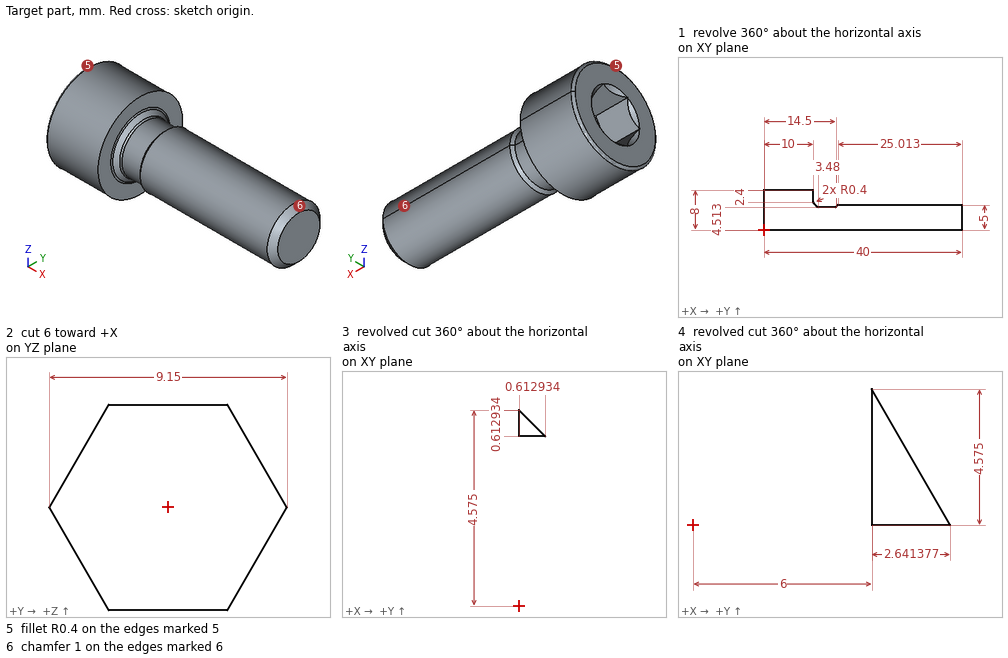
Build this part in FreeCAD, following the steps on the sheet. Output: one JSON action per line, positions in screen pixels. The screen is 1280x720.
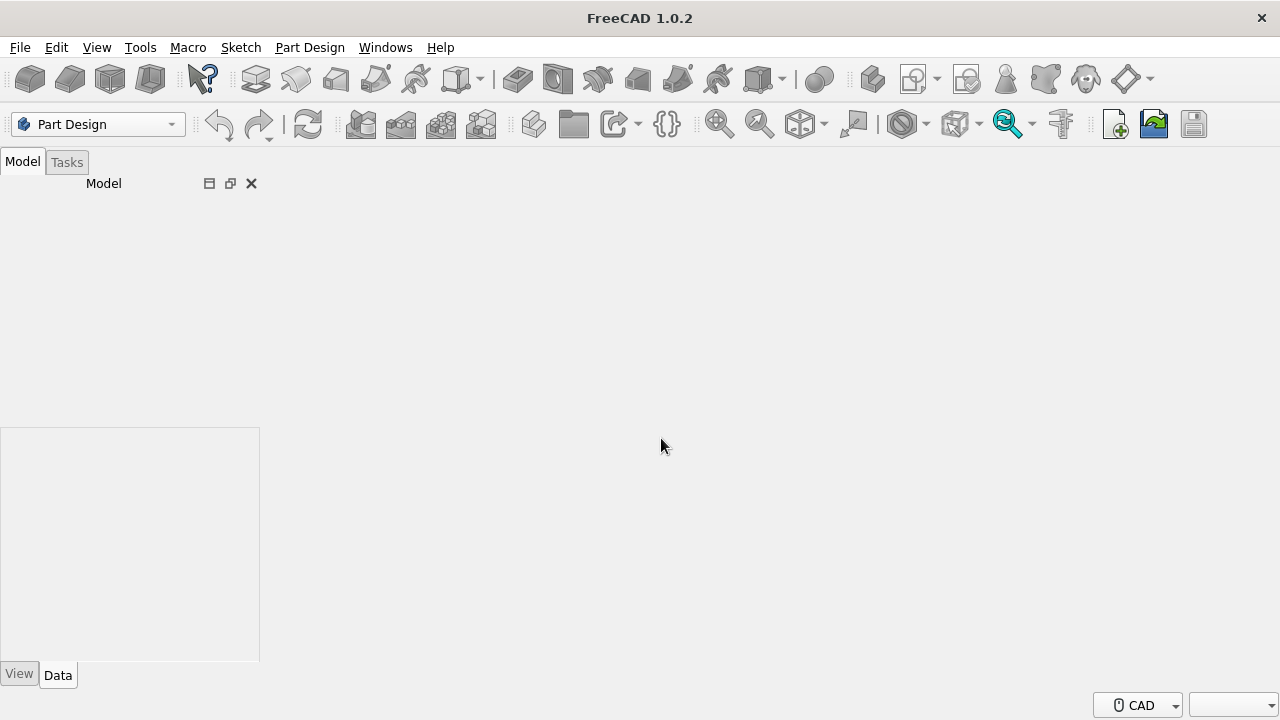
{"action": "left_click", "coordinate": [1114, 124]}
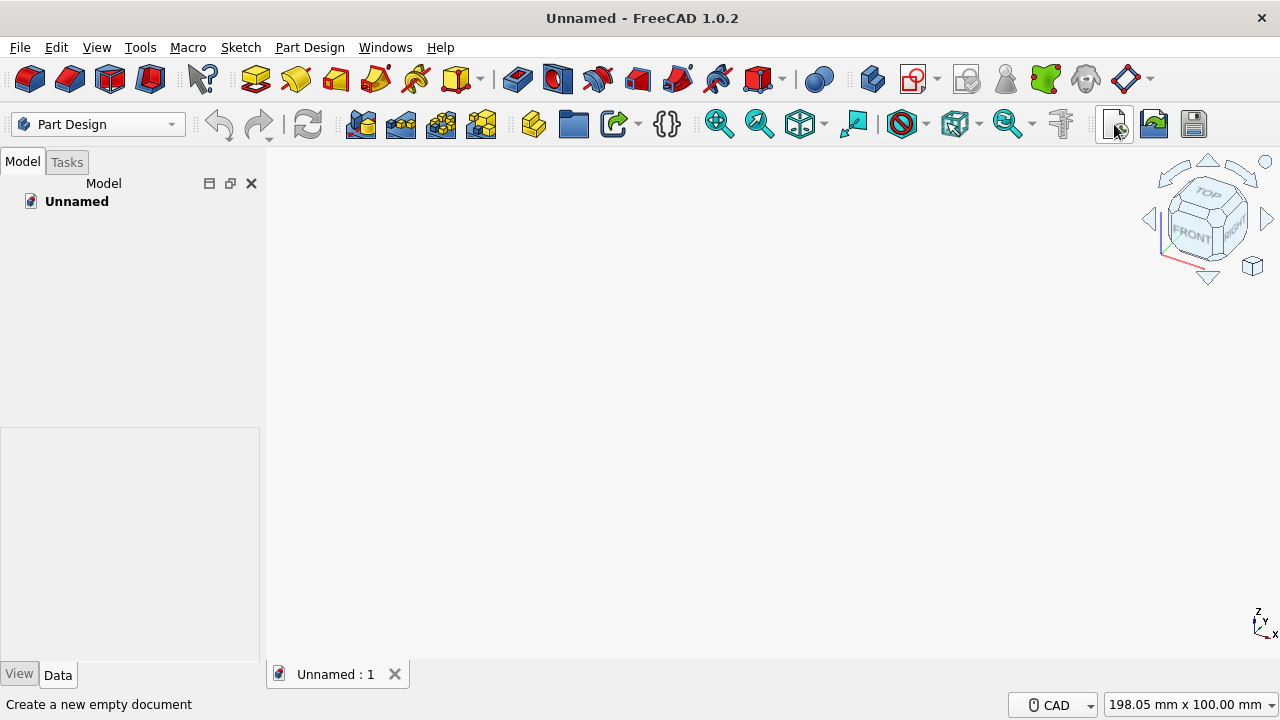
{"action": "left_click", "coordinate": [914, 80]}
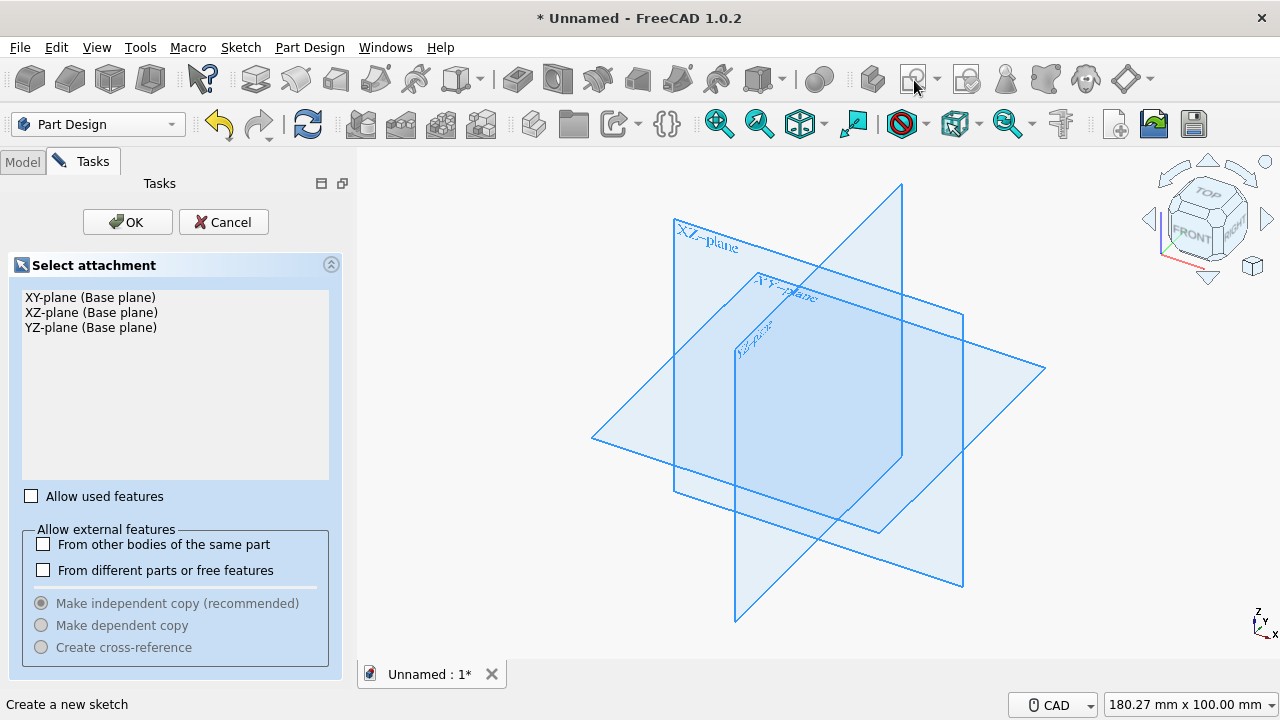
{"action": "left_click", "coordinate": [82, 298]}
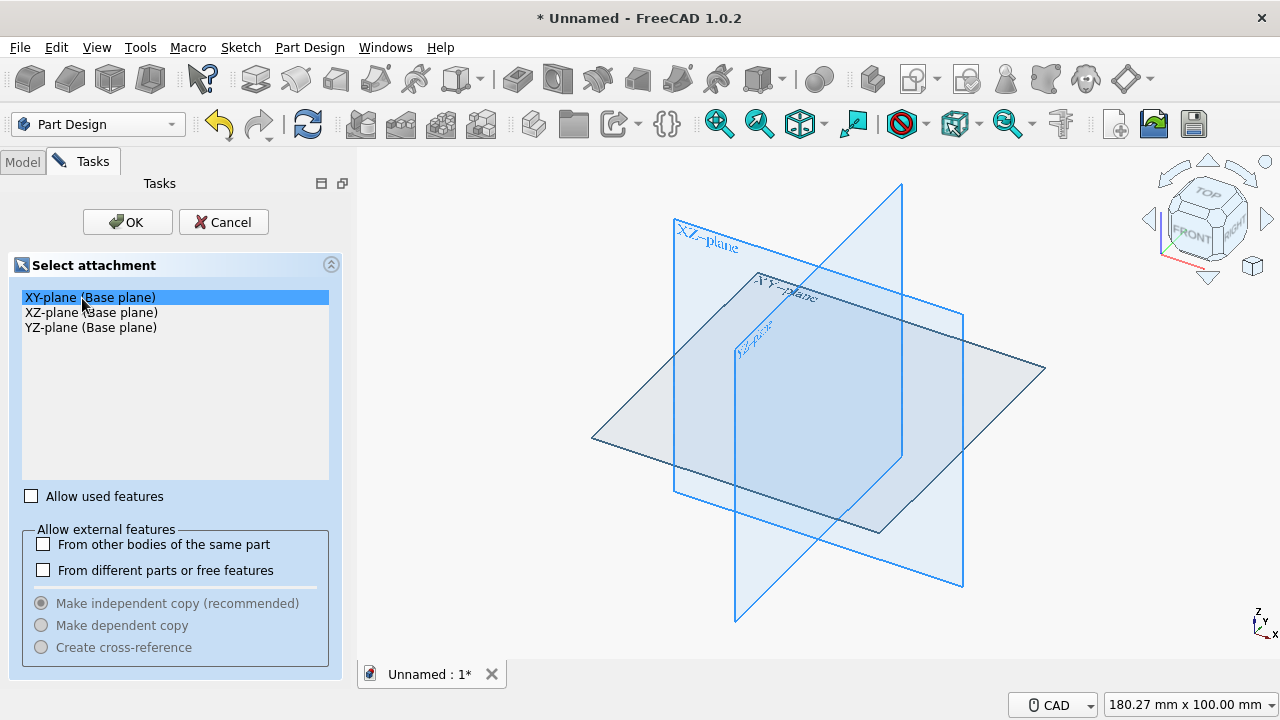
{"action": "left_click", "coordinate": [128, 222]}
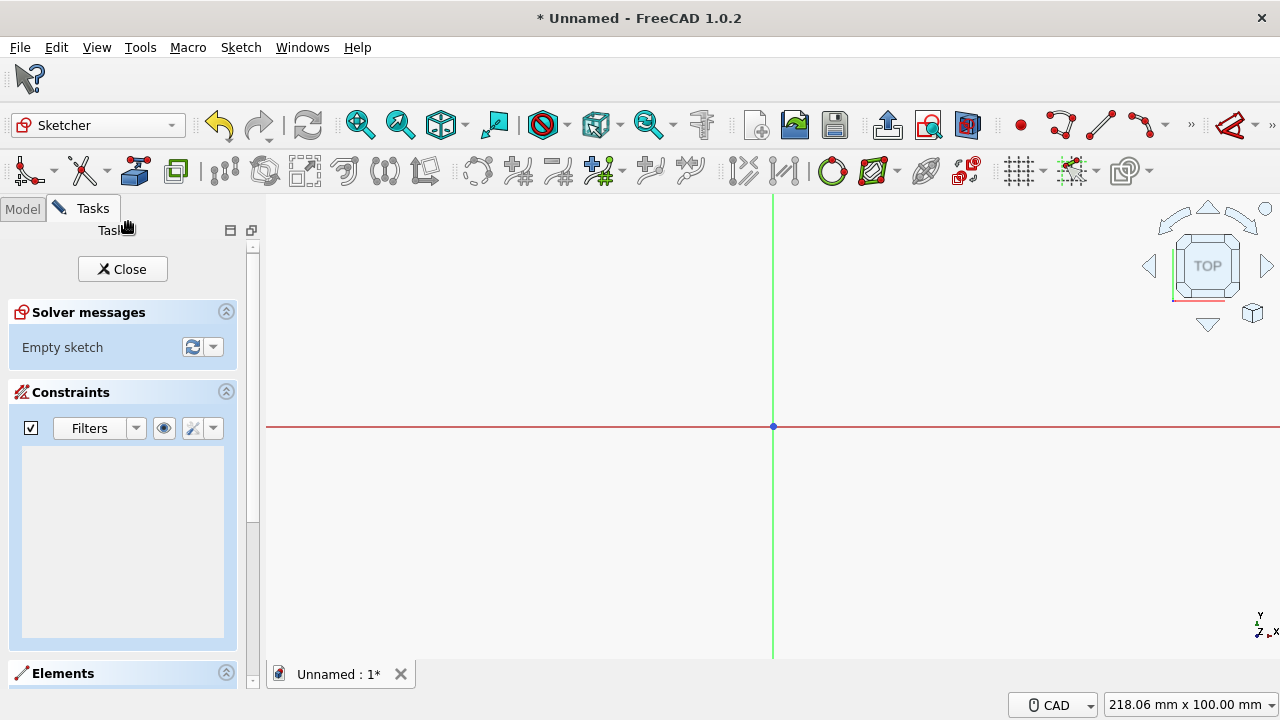
{"action": "scroll", "coordinate": [936, 400], "scroll_direction": "up", "scroll_amount": 6}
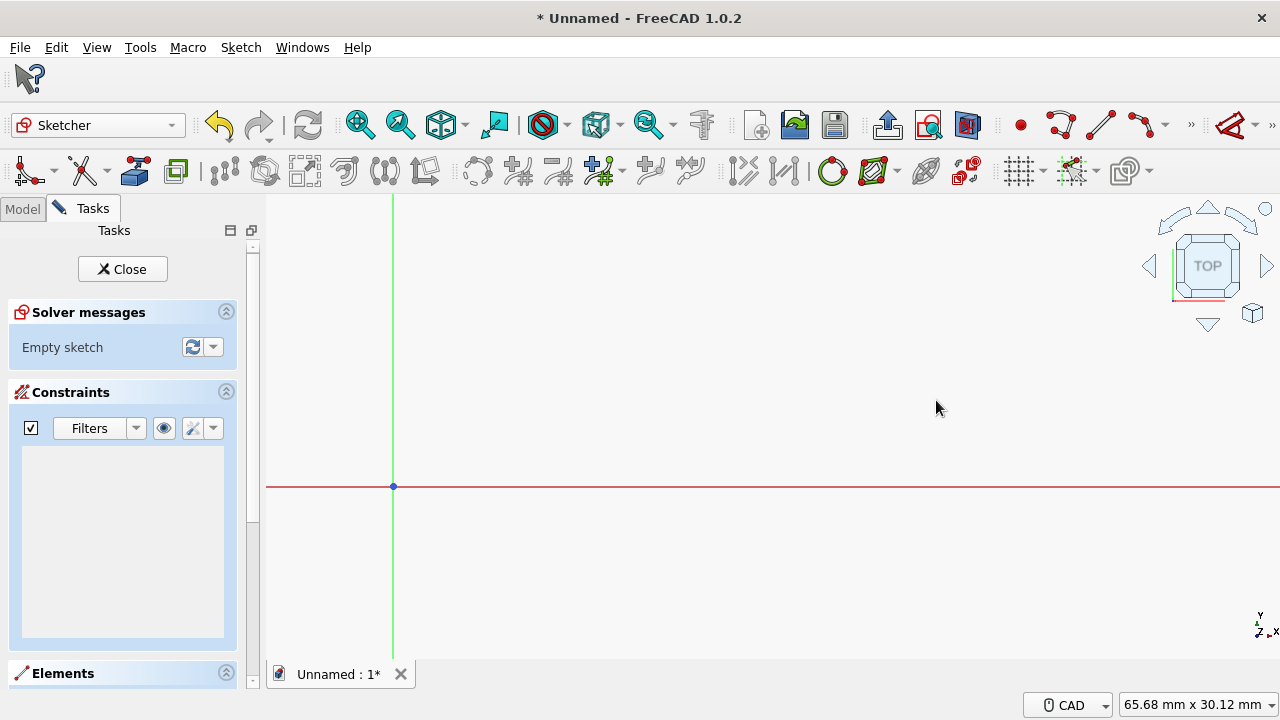
{"action": "left_click", "coordinate": [1102, 126]}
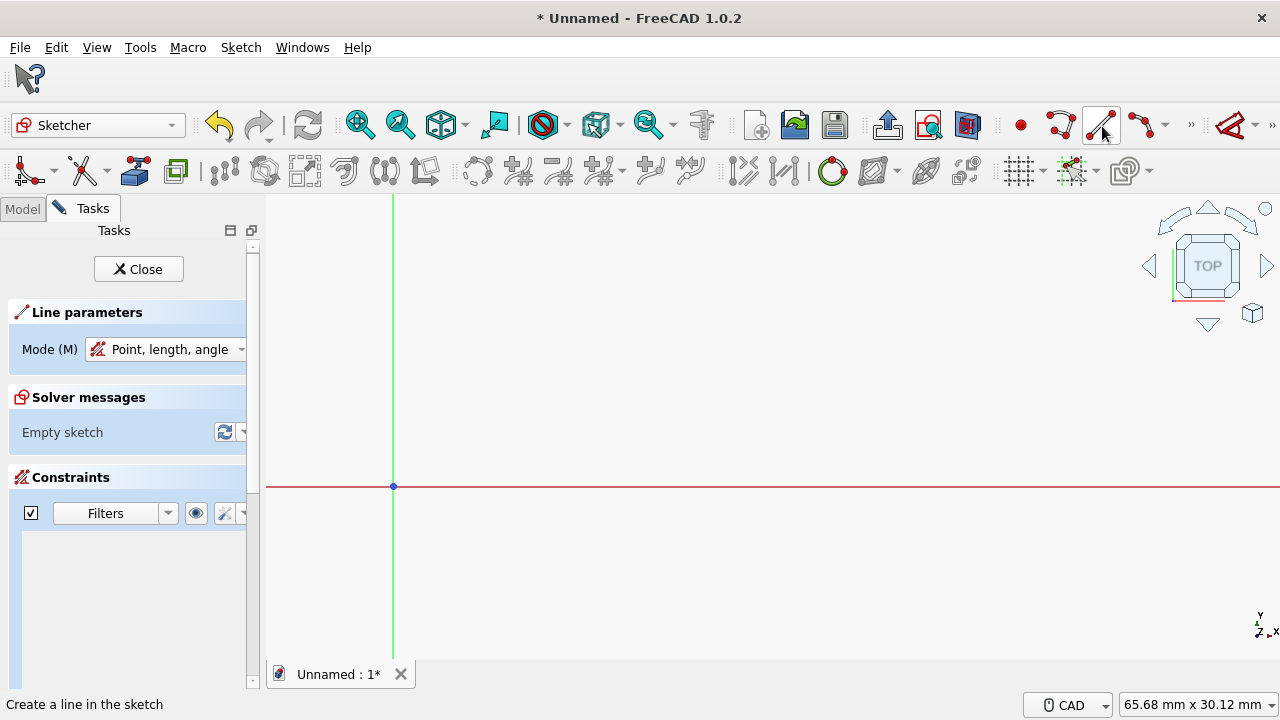
{"action": "left_click", "coordinate": [559, 415]}
{"action": "left_click", "coordinate": [549, 405]}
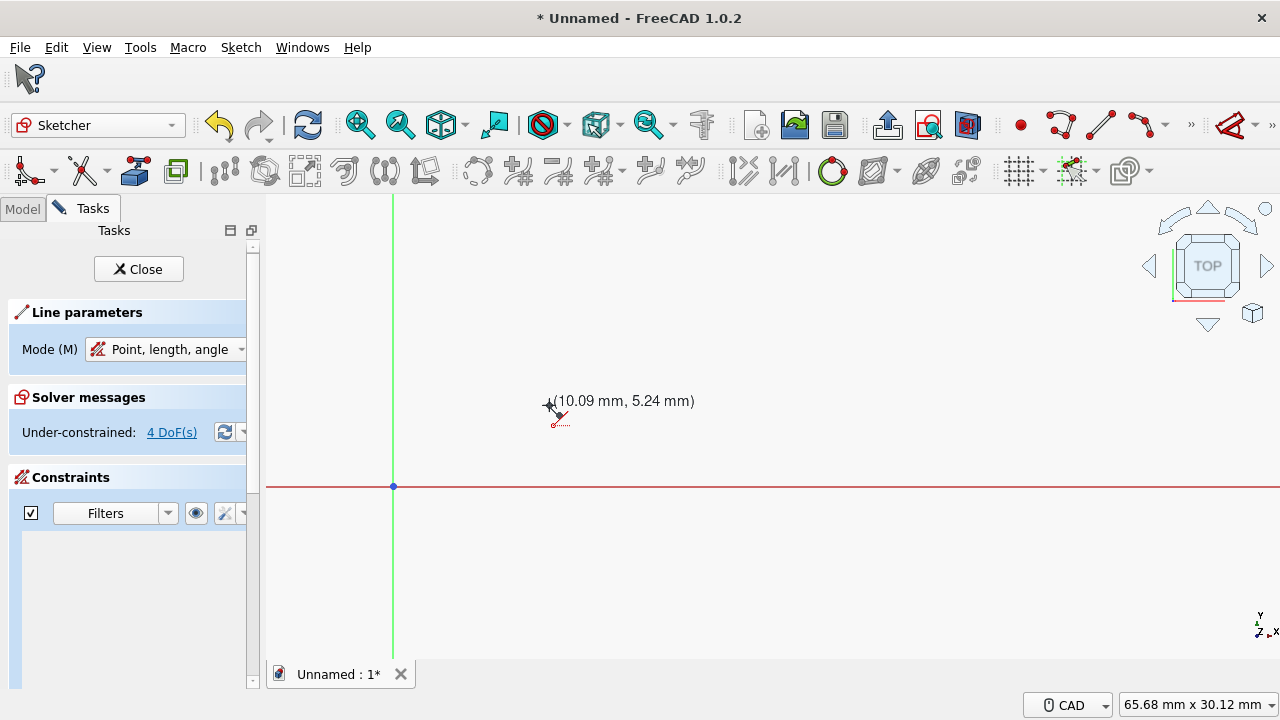
{"action": "left_click", "coordinate": [1062, 126]}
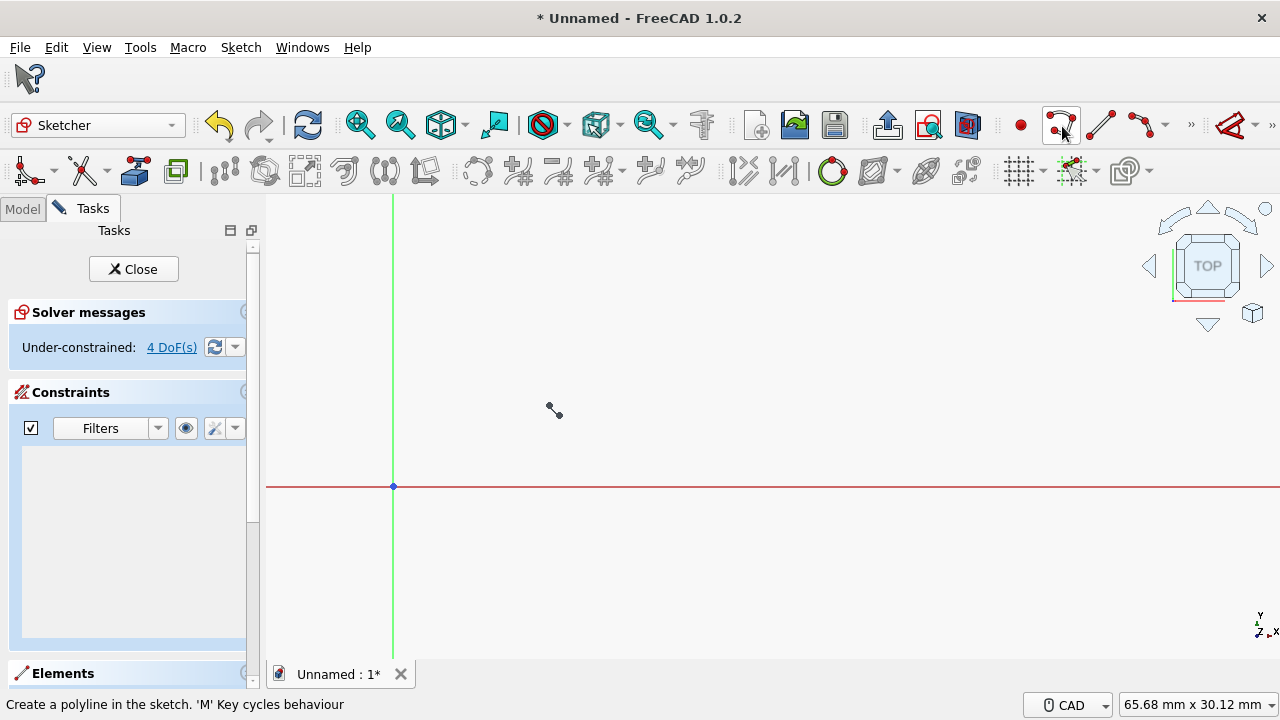
{"action": "scroll", "coordinate": [548, 400], "scroll_direction": "up", "scroll_amount": 7}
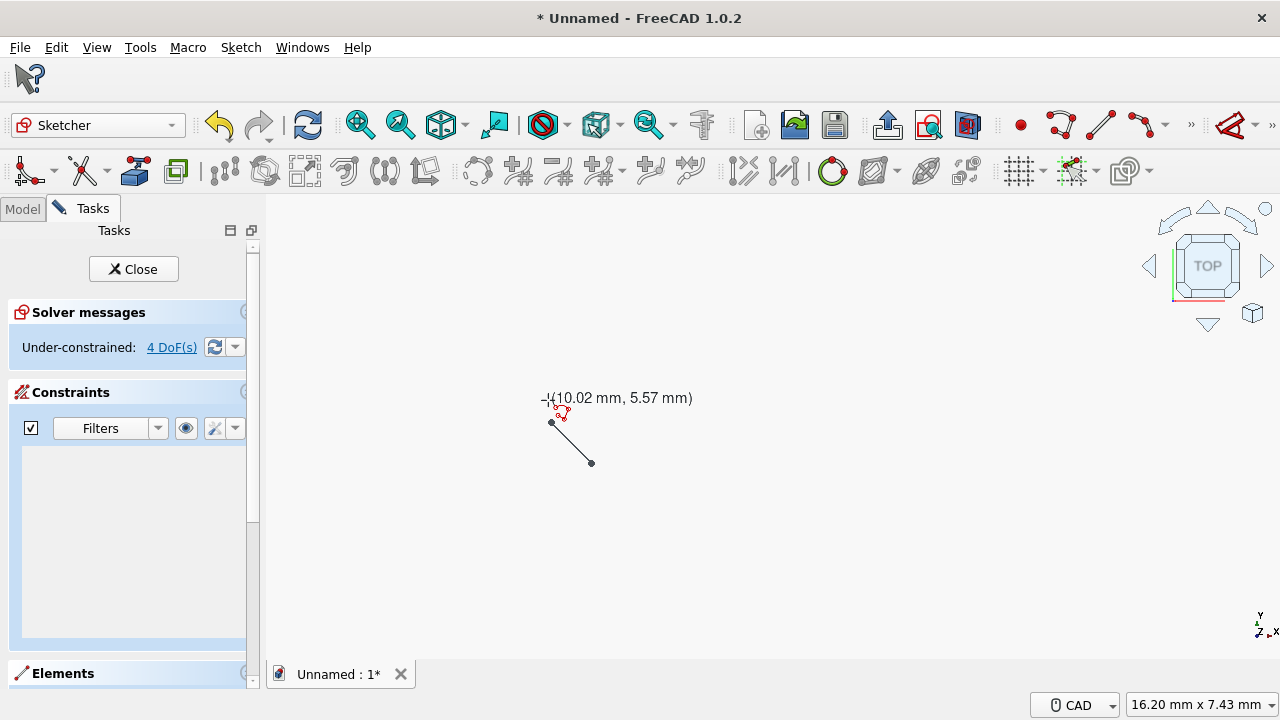
{"action": "left_click", "coordinate": [546, 401]}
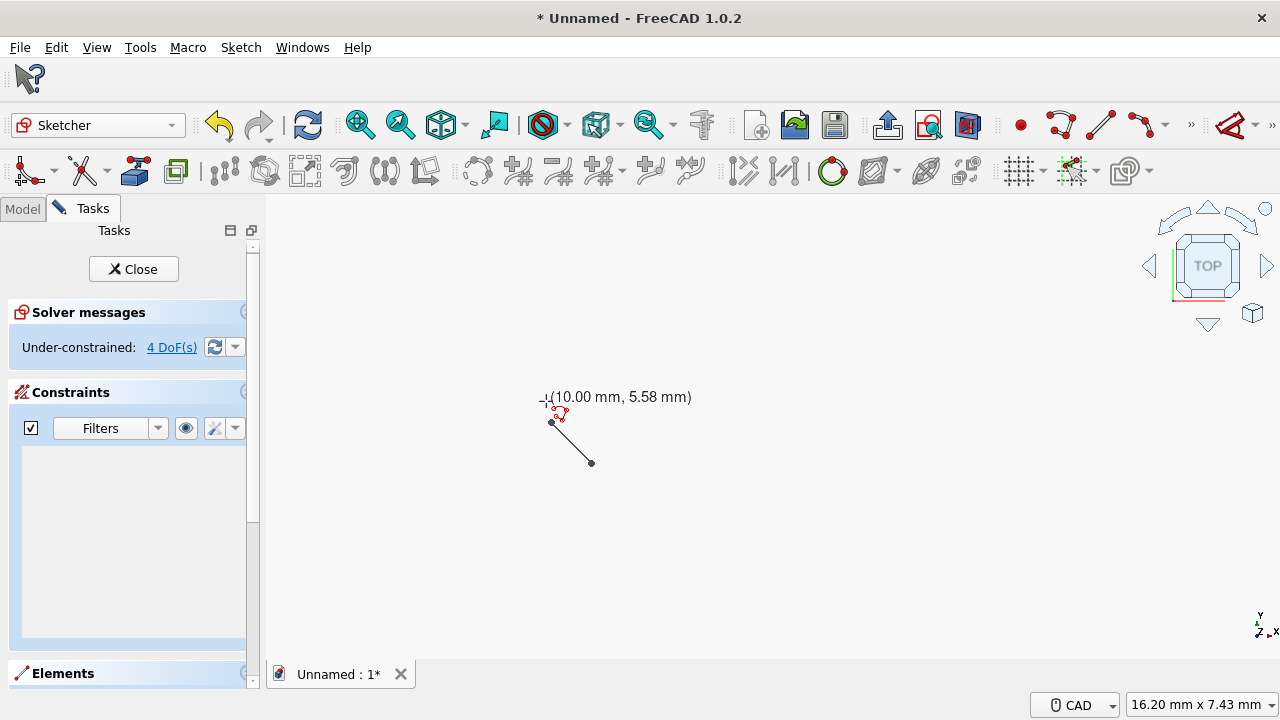
{"action": "scroll", "coordinate": [552, 402], "scroll_direction": "down", "scroll_amount": 7}